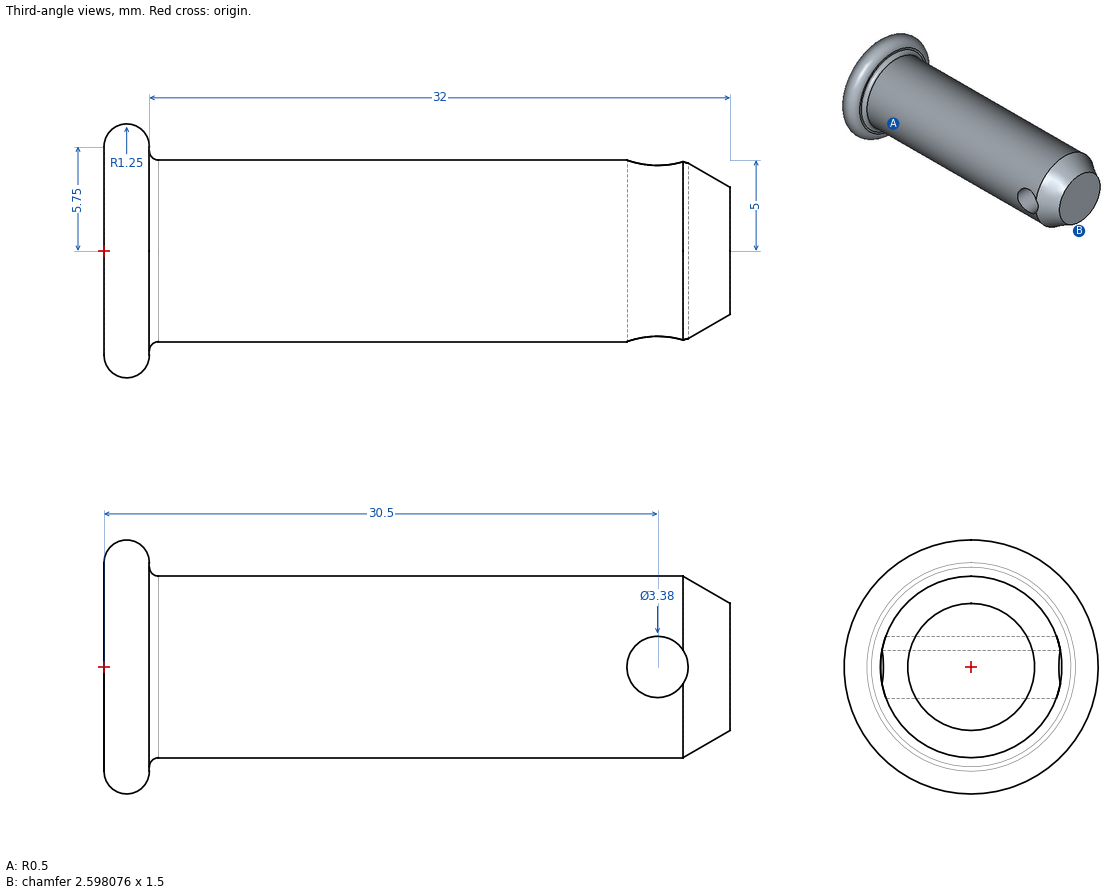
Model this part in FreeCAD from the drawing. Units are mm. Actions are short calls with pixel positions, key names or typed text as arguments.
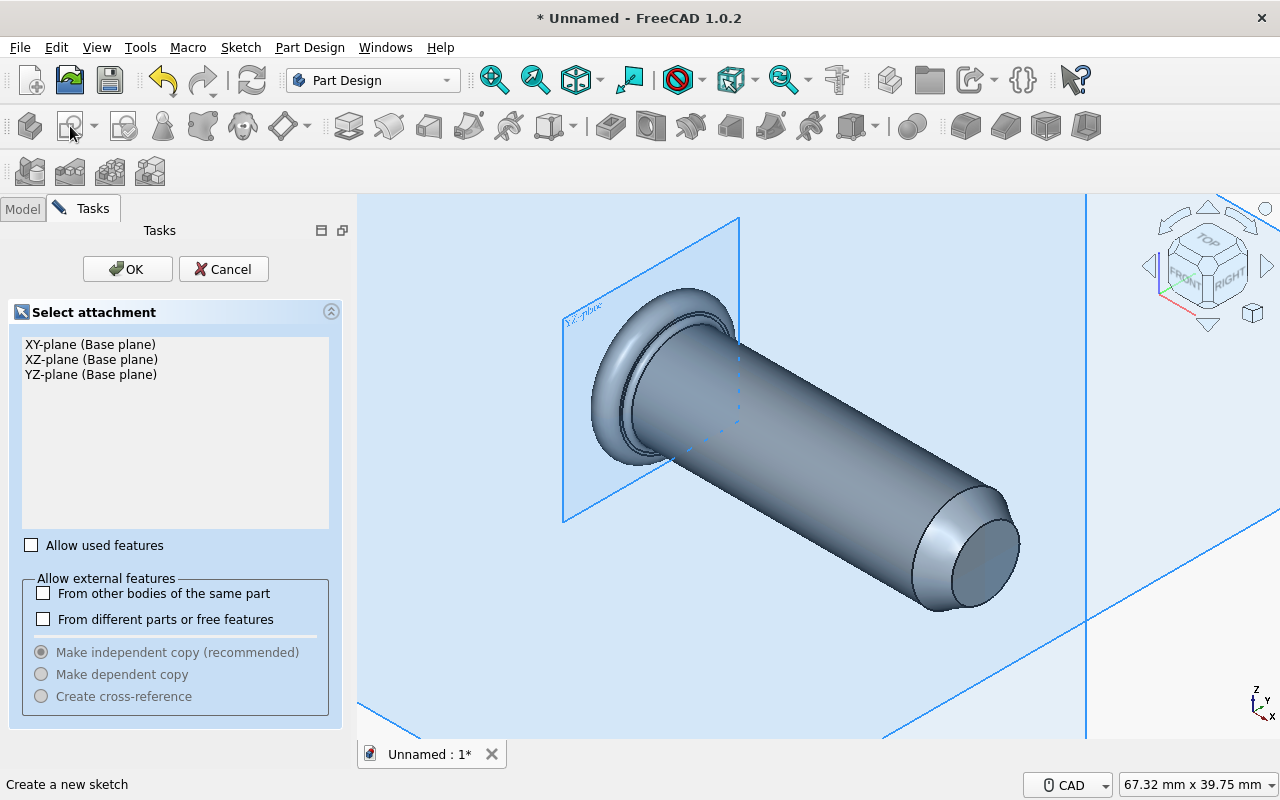
click(82, 360)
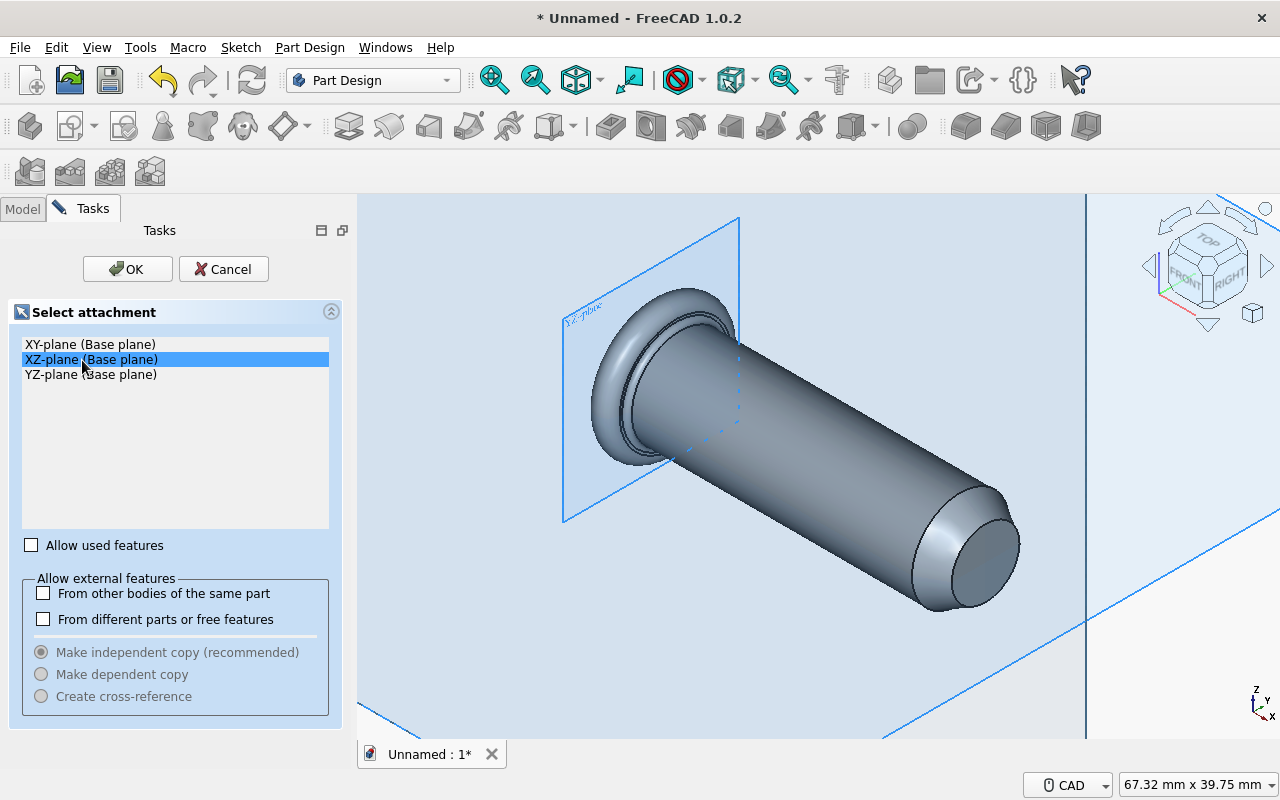
click(128, 269)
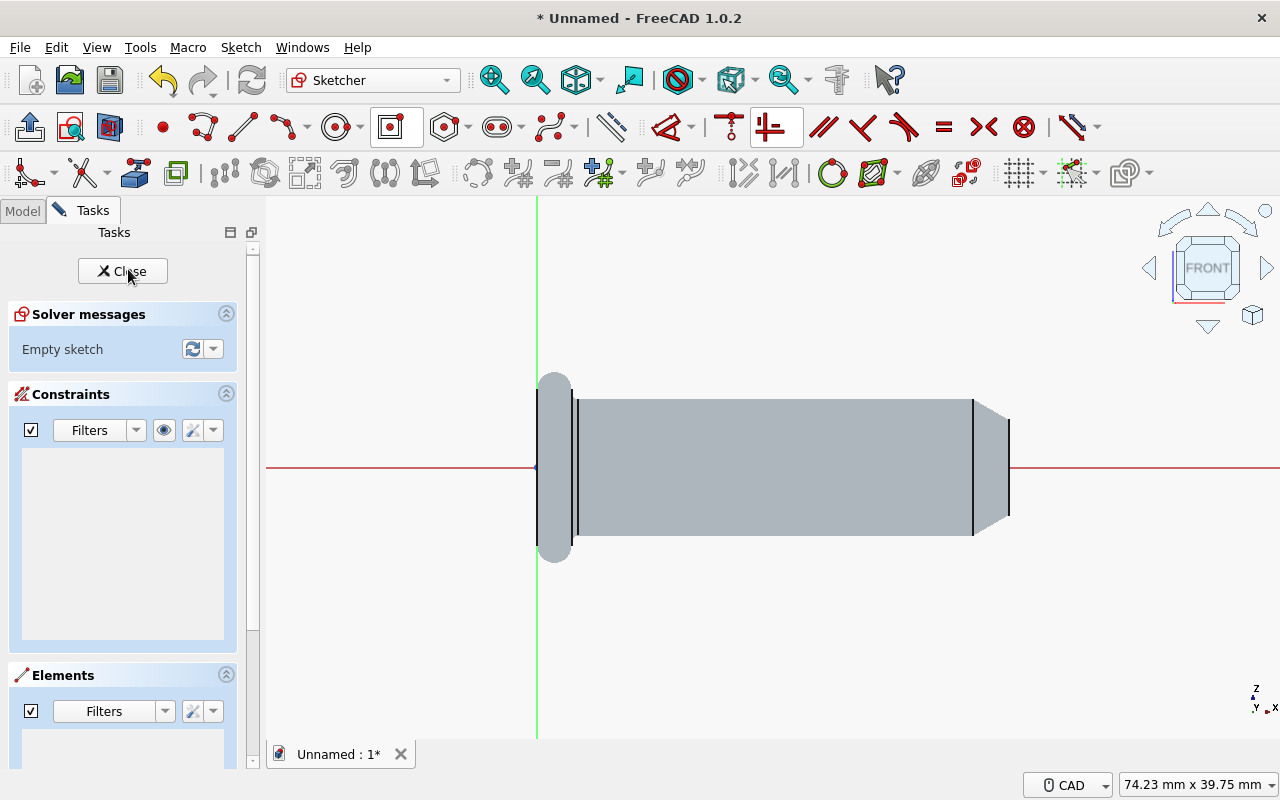
click(110, 128)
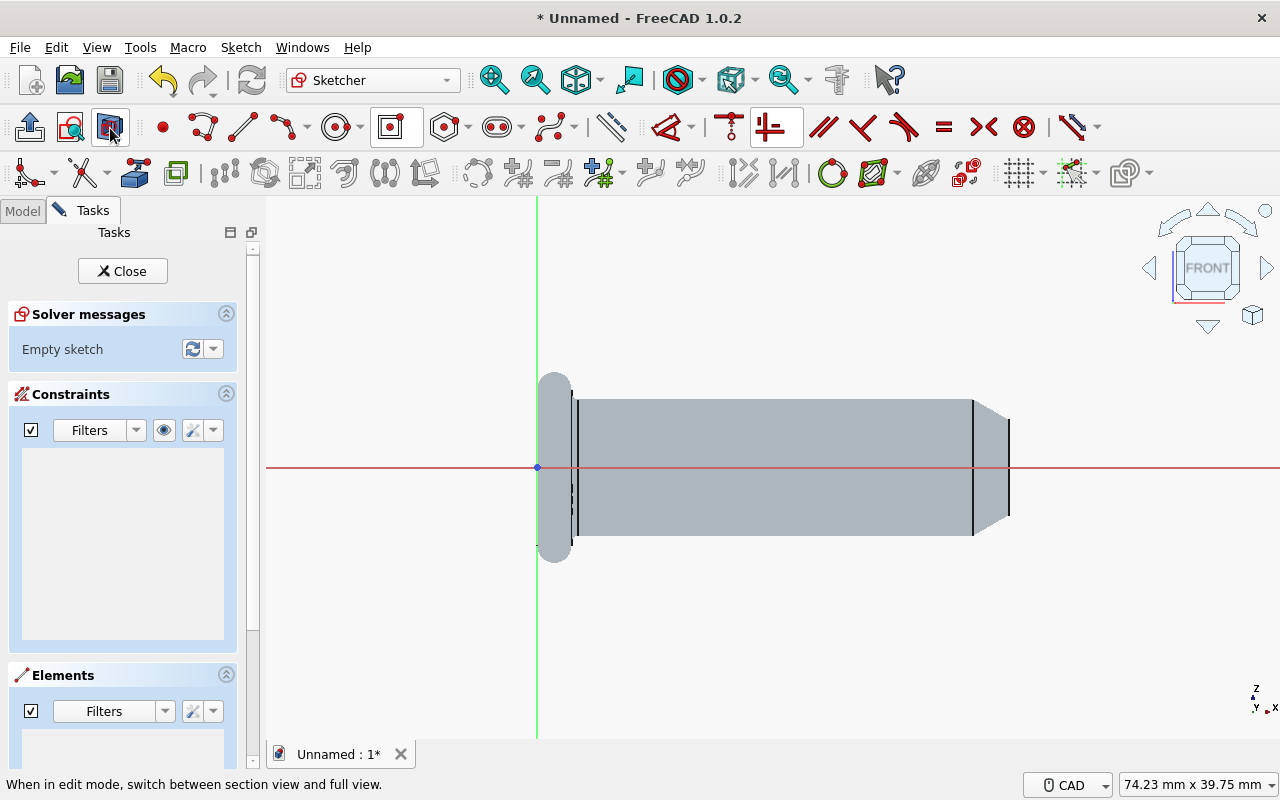
scroll(993, 468, up, 10)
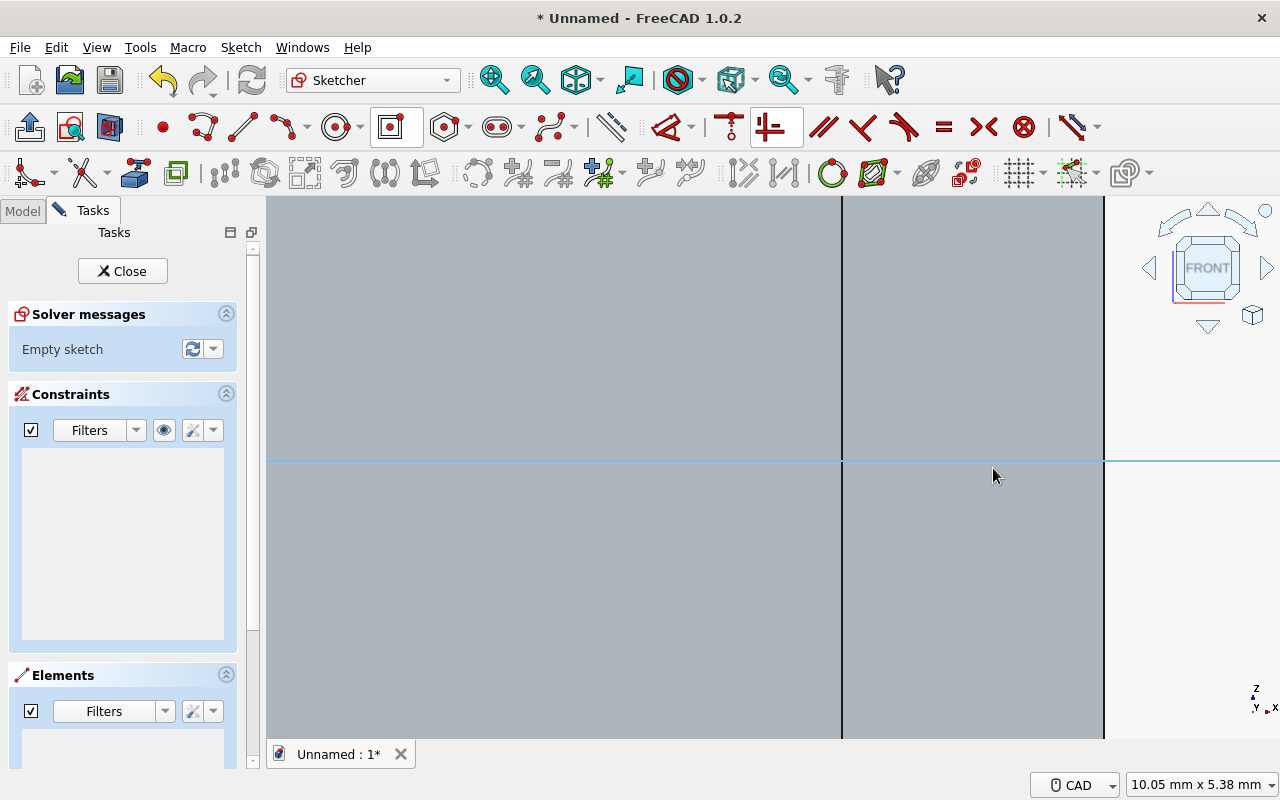
key(g)
key(c)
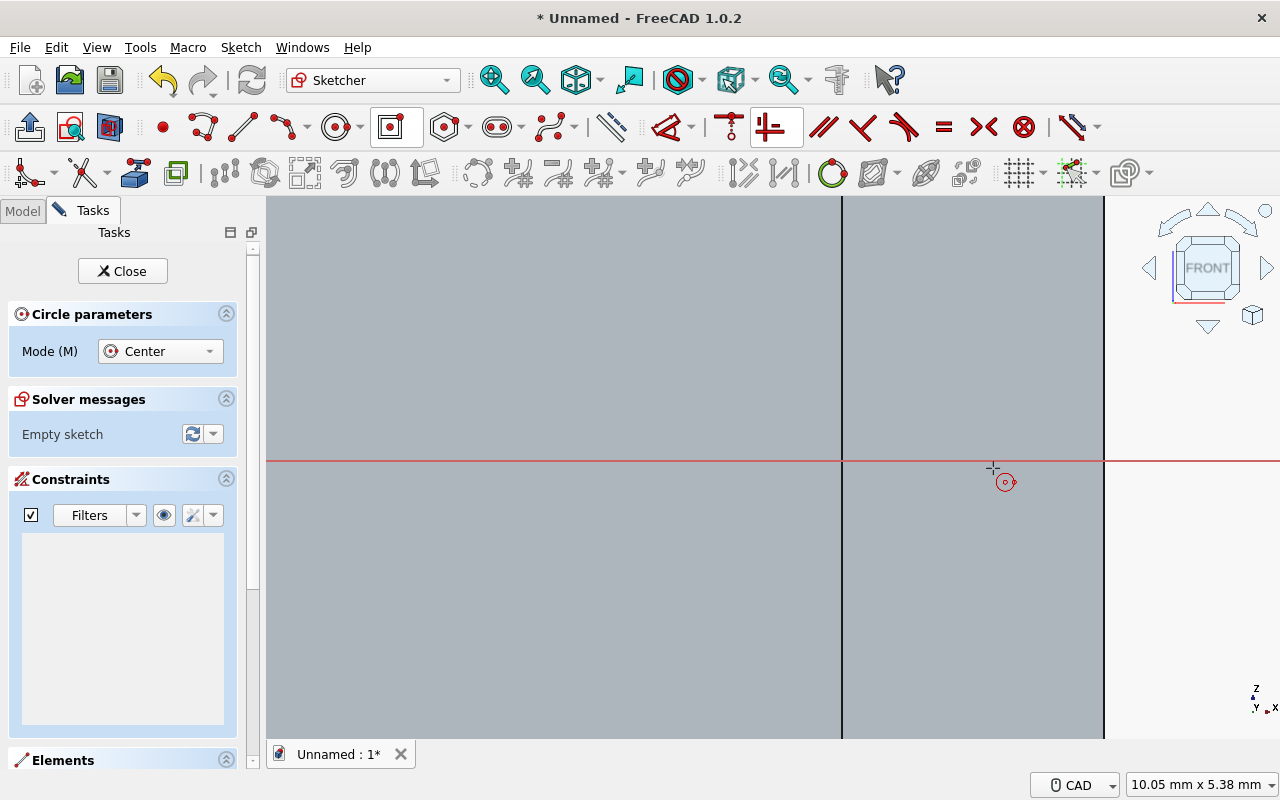
click(700, 461)
click(821, 340)
key(Escape)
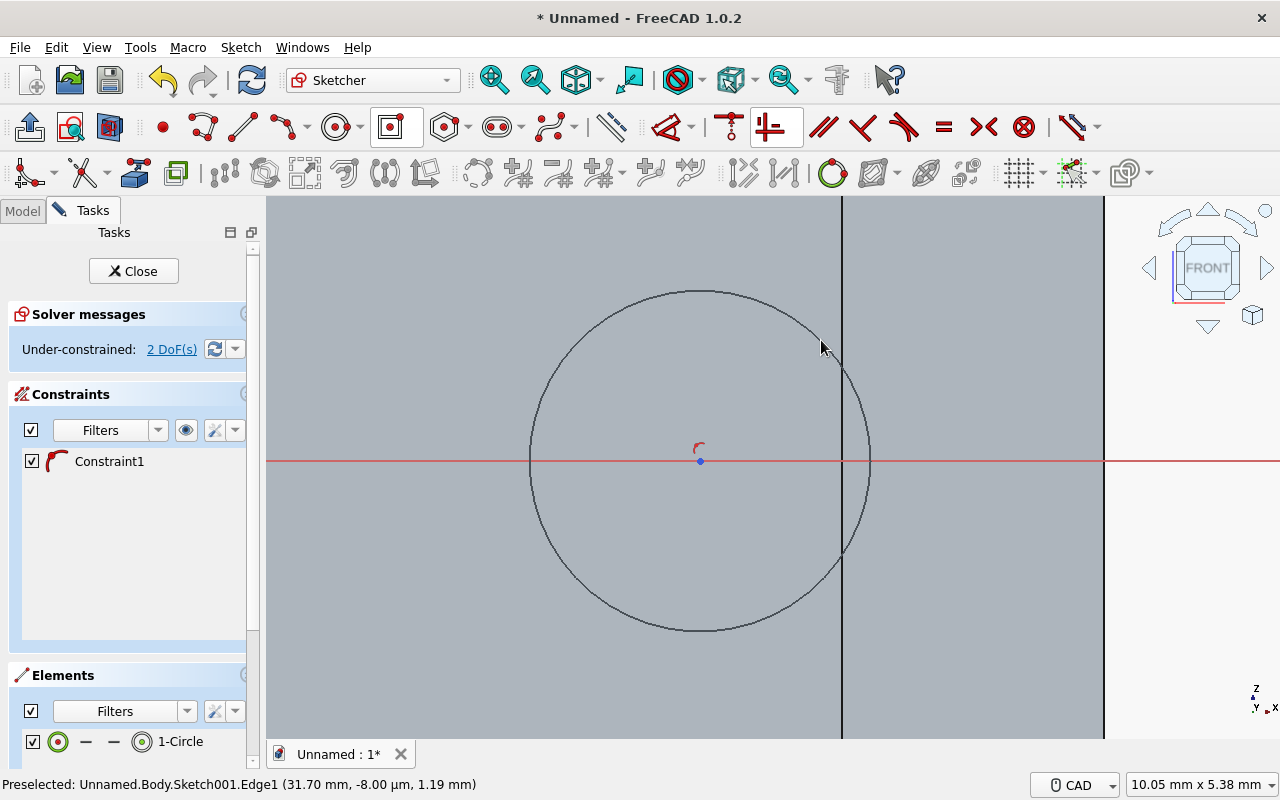
click(820, 340)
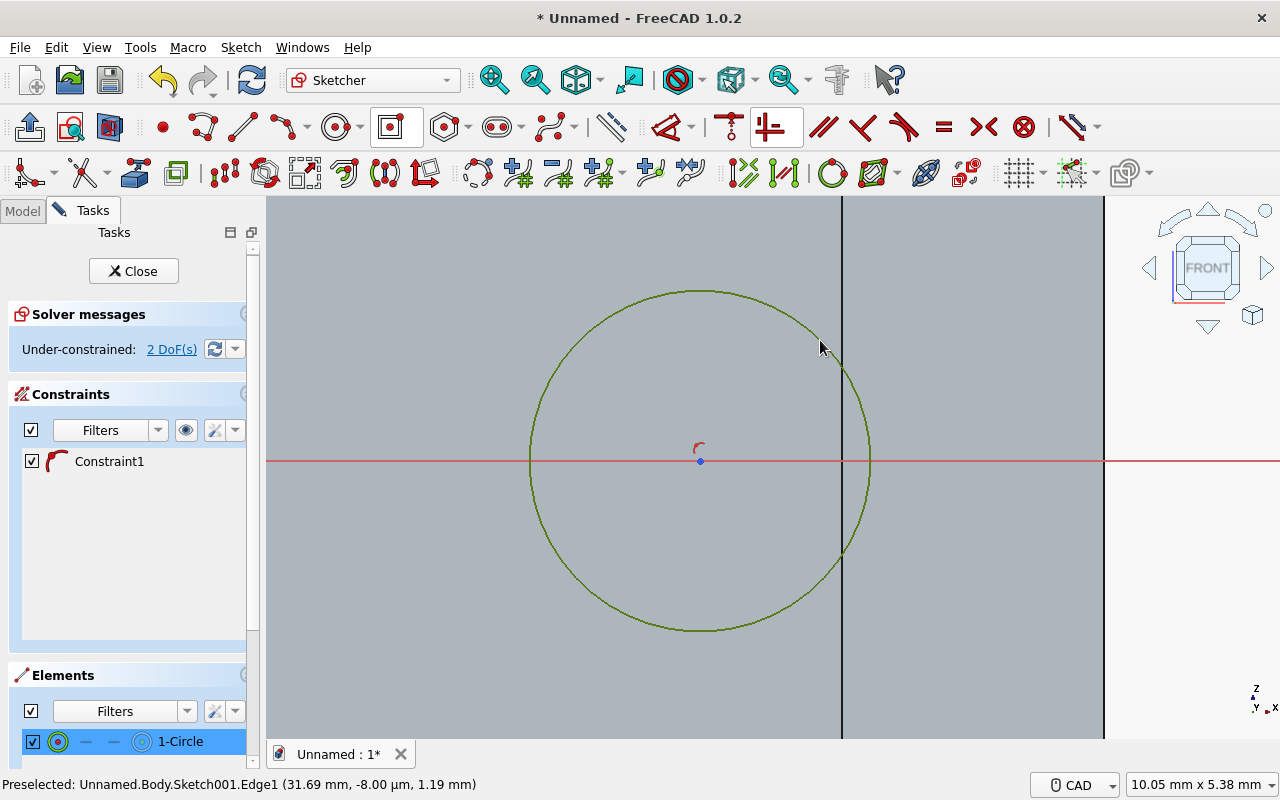
click(694, 128)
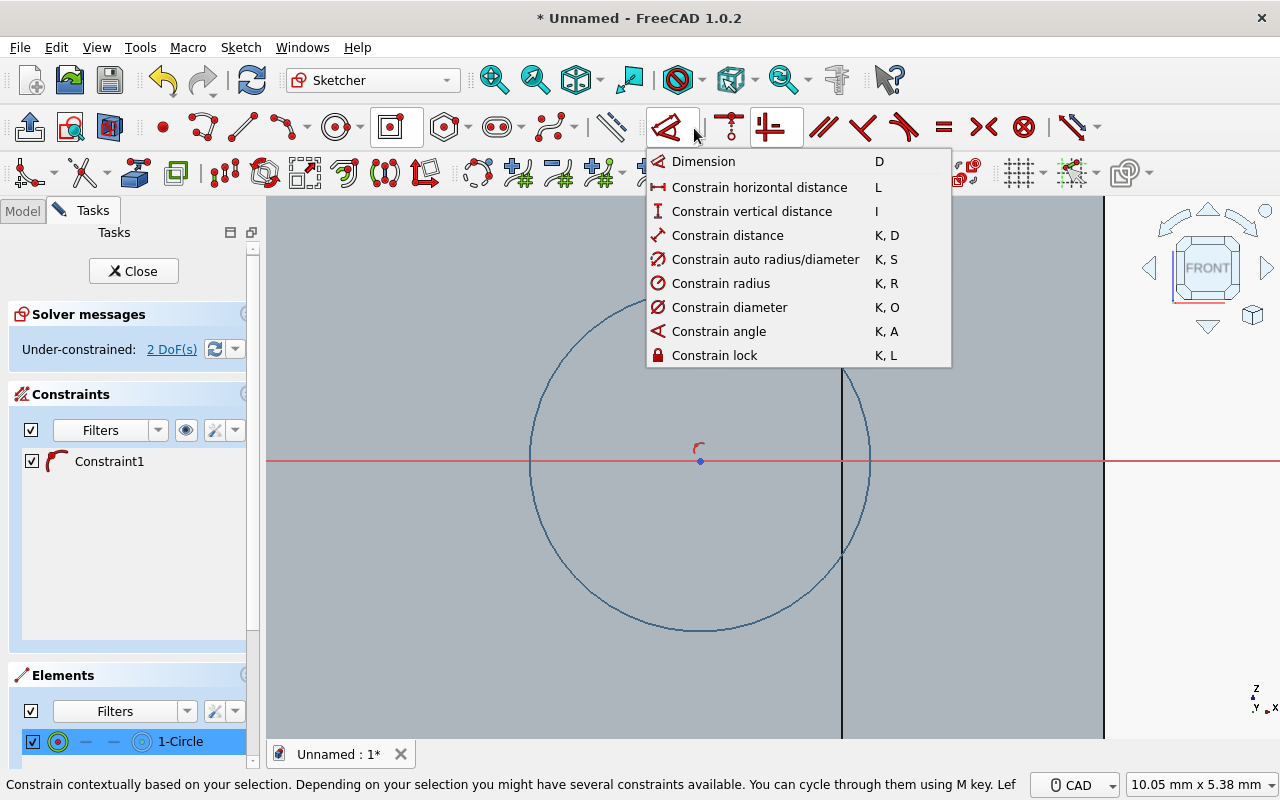
click(799, 307)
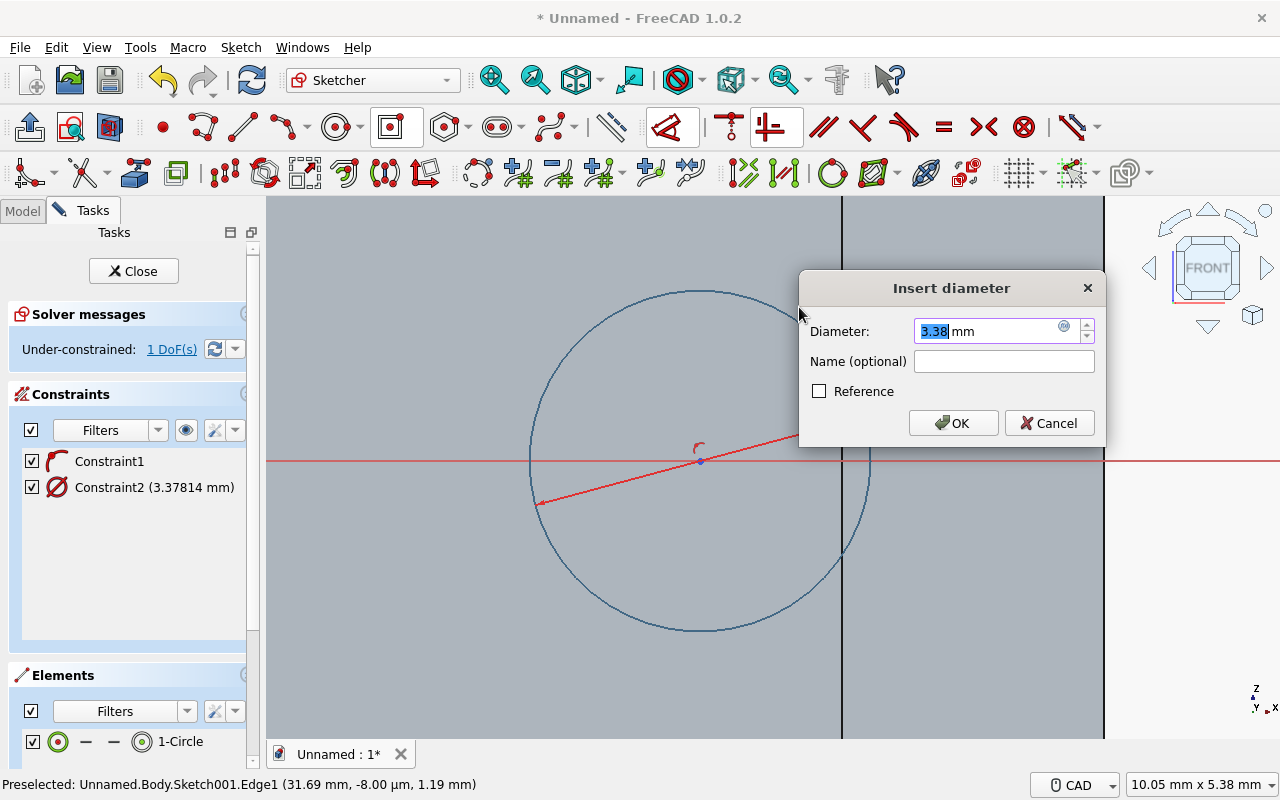
text(3.38)
key(Return)